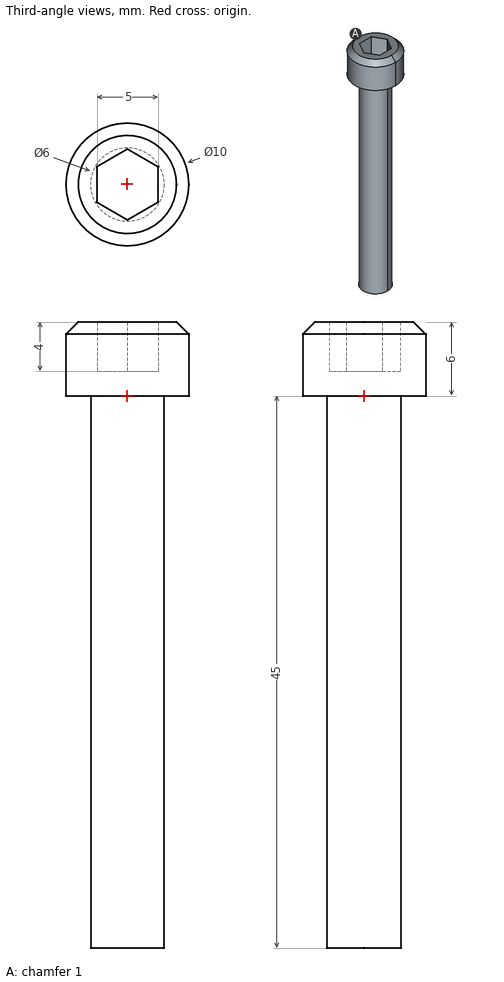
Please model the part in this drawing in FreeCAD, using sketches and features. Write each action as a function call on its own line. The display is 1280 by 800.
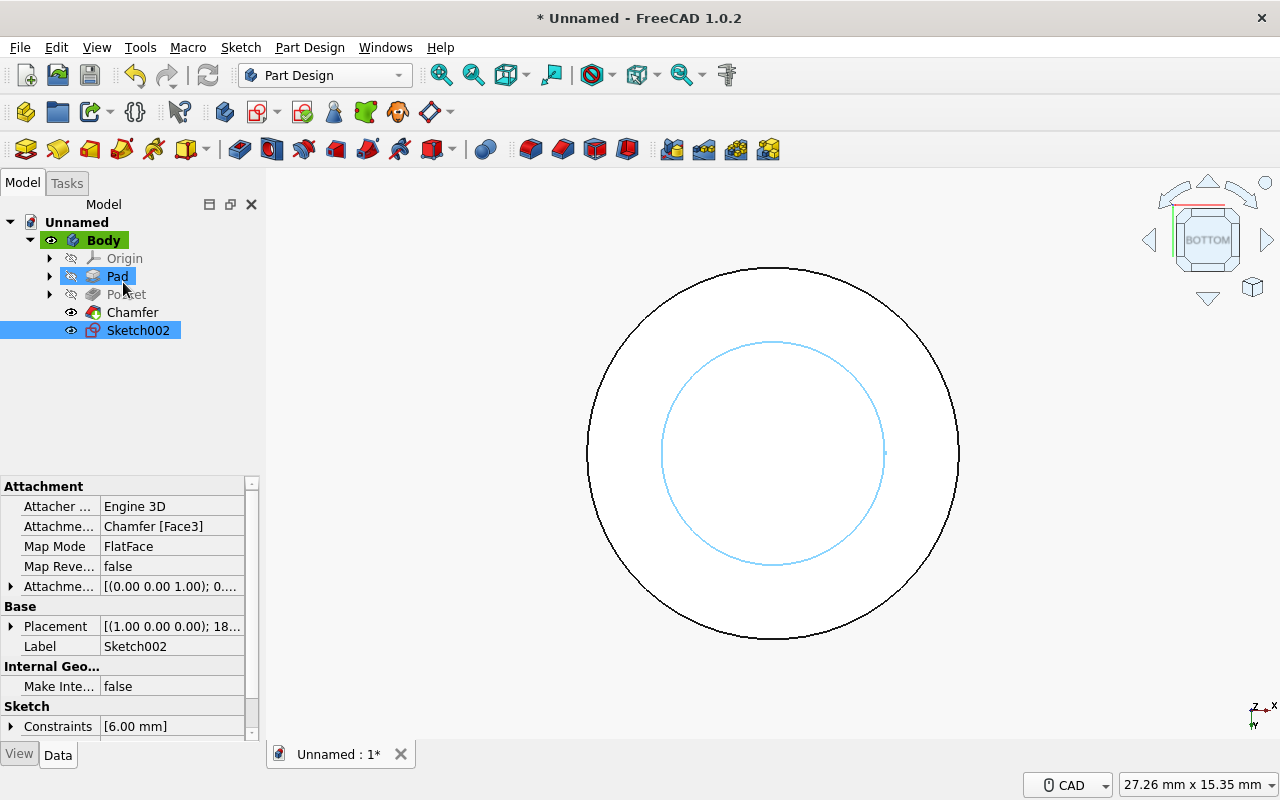
click(26, 150)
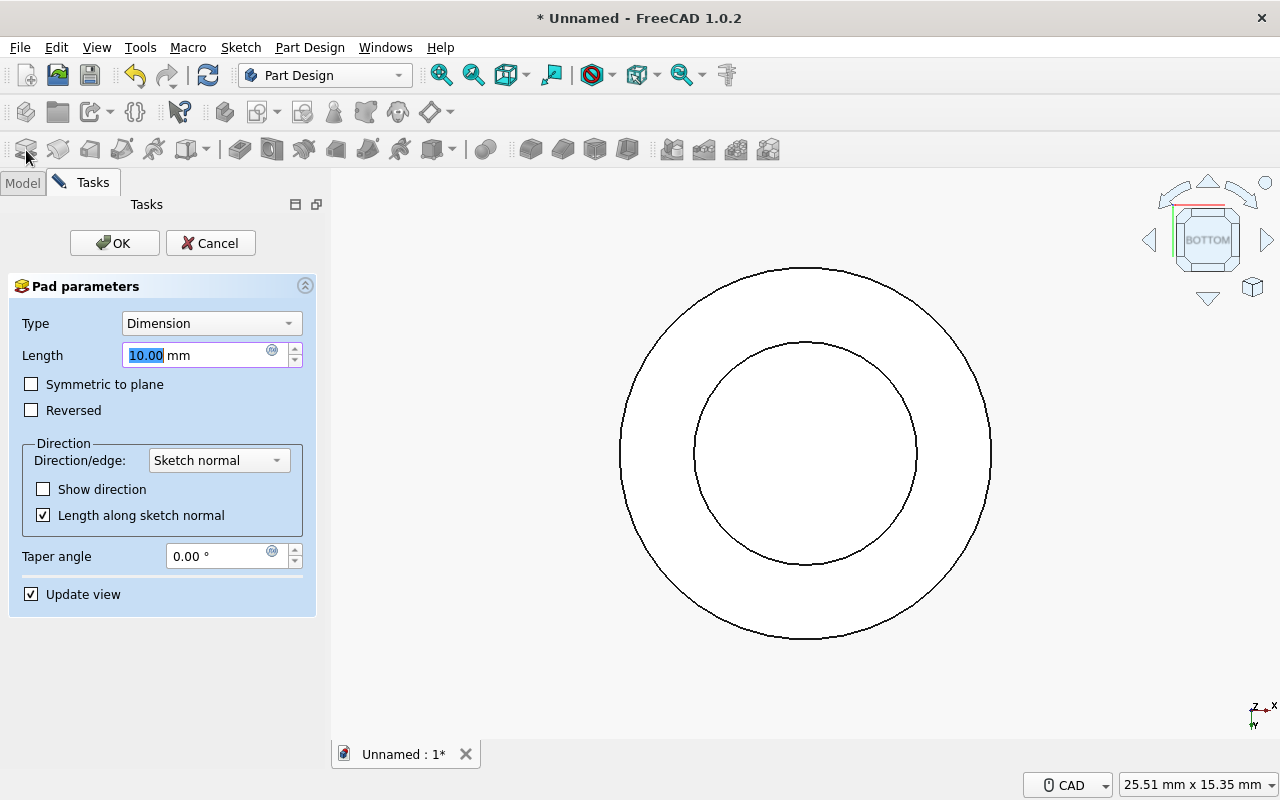
text(45)
key(Tab)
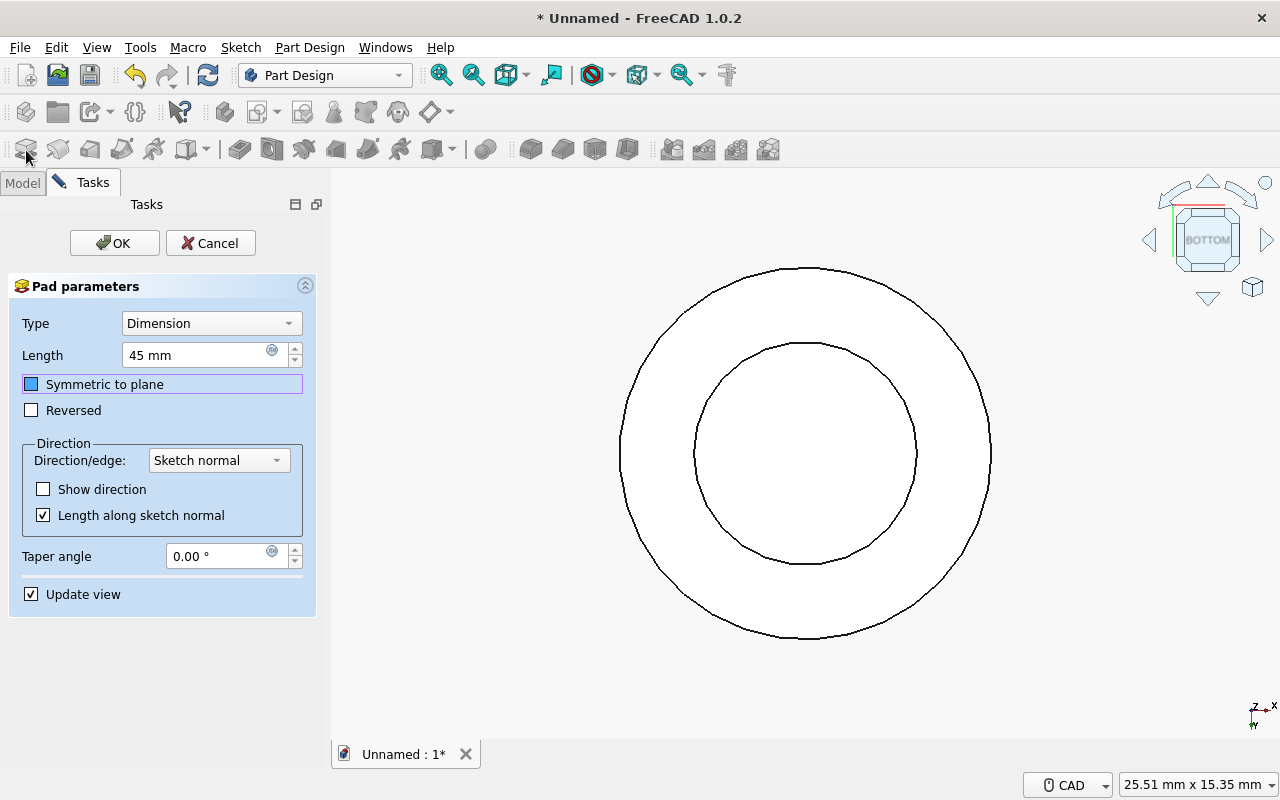
click(115, 243)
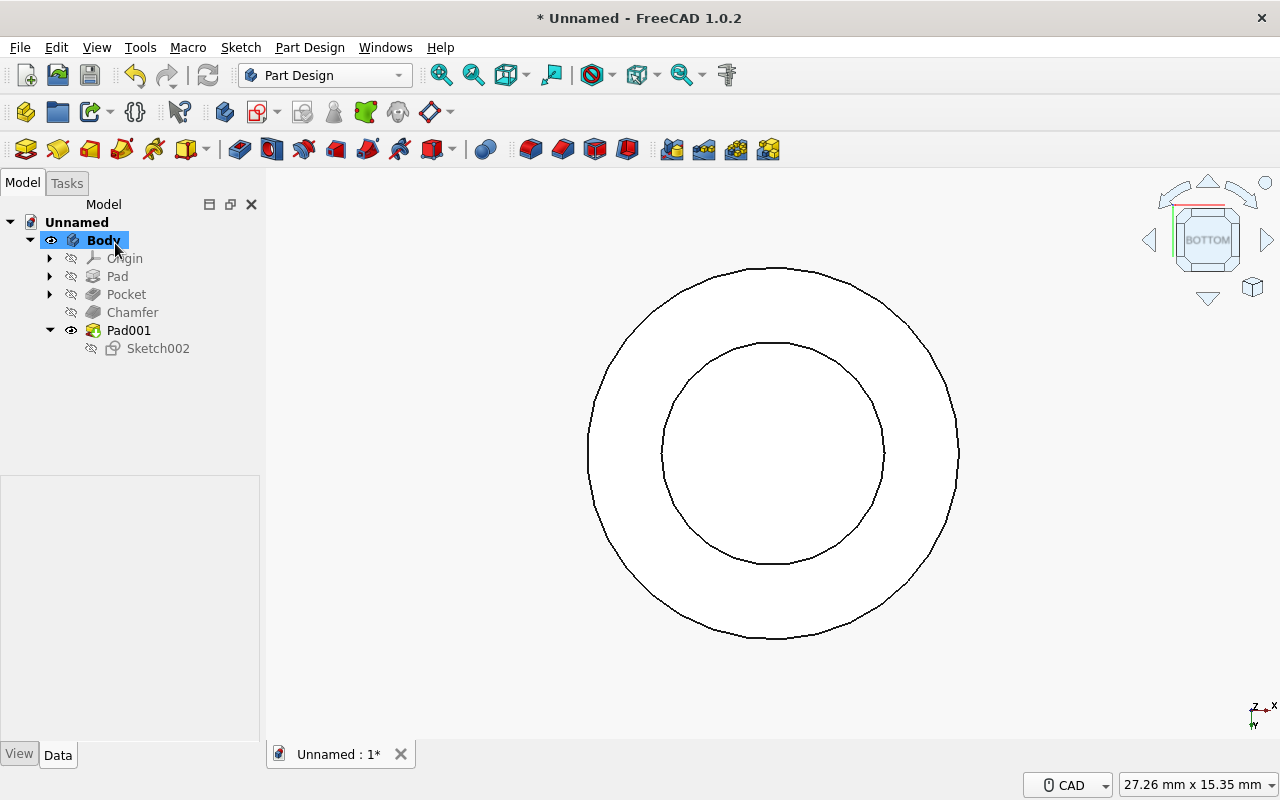
key(0)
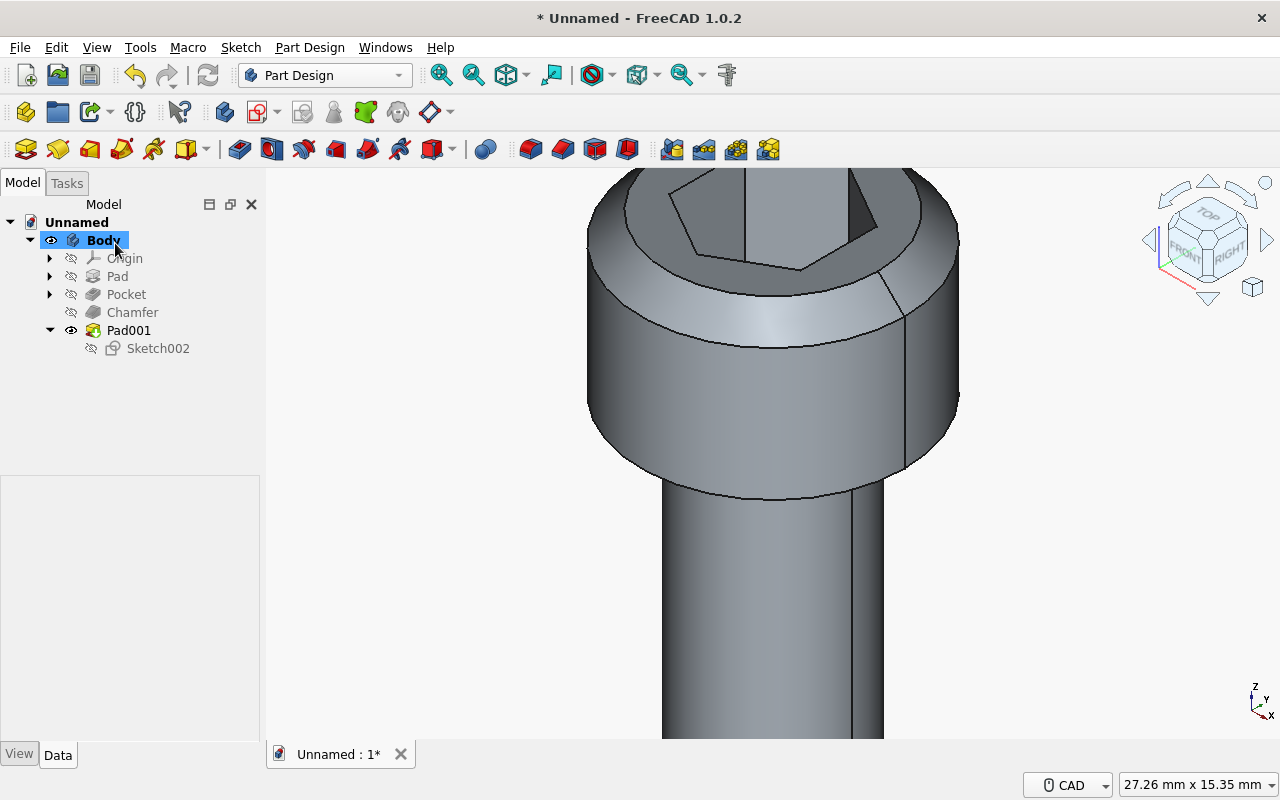
click(442, 76)